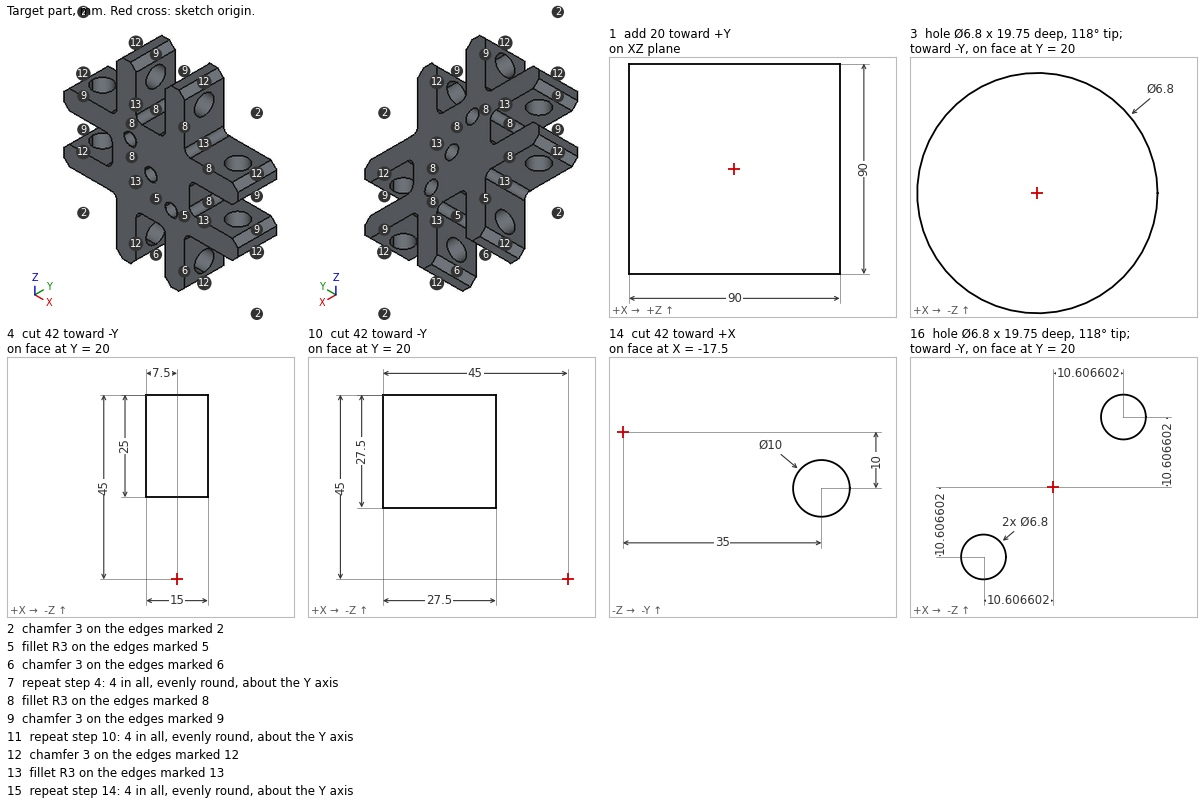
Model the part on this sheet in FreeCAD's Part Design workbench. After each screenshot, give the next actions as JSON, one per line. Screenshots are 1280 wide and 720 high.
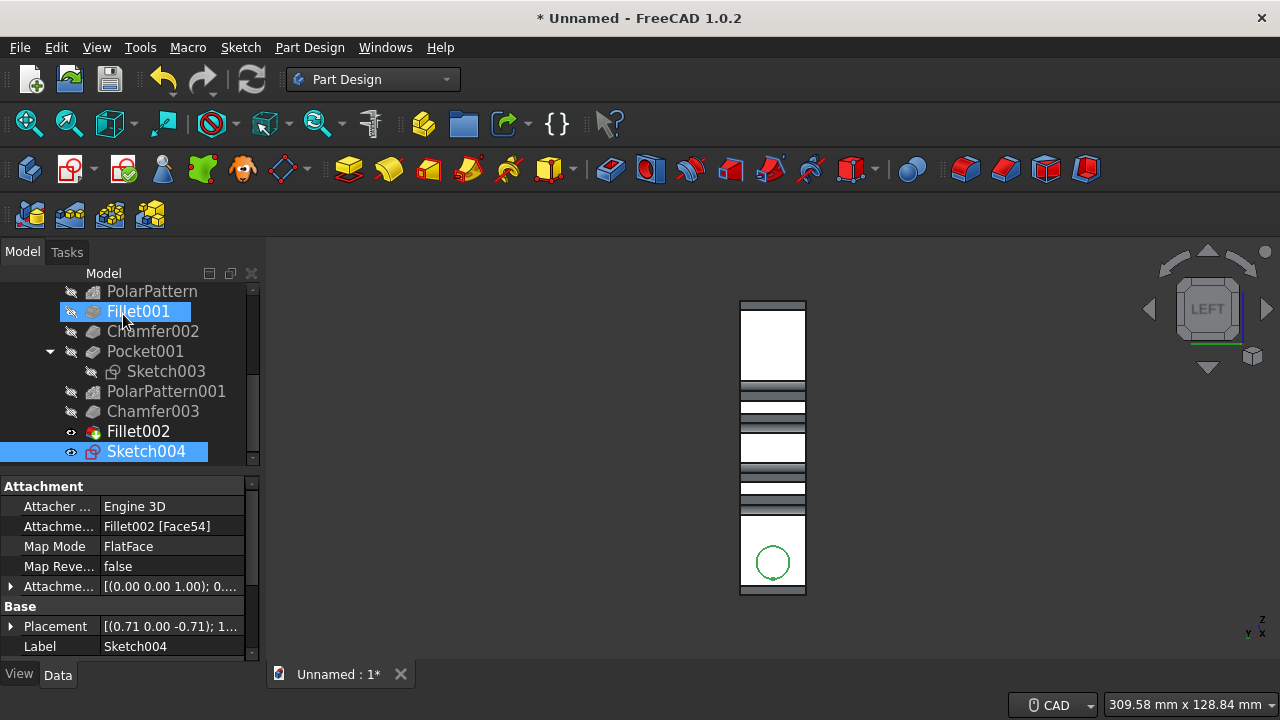
{"action": "left_click", "coordinate": [612, 170]}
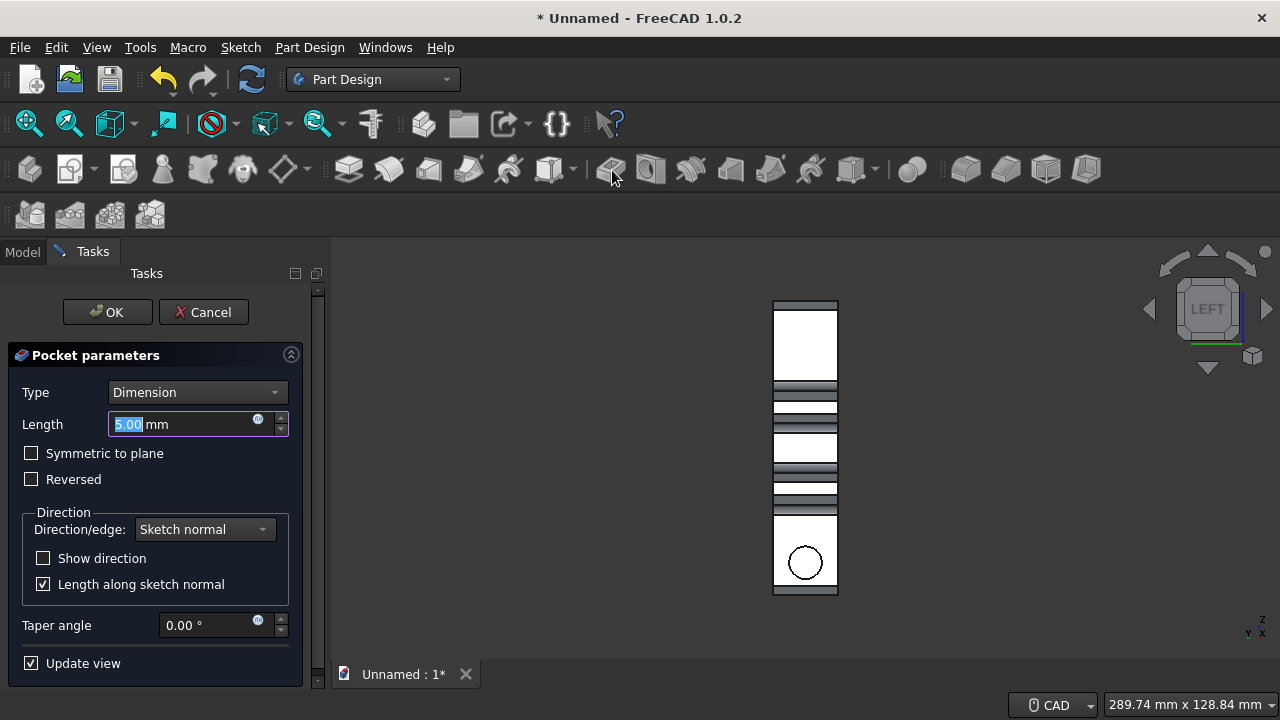
{"action": "type", "text": "42"}
{"action": "key", "text": "Tab"}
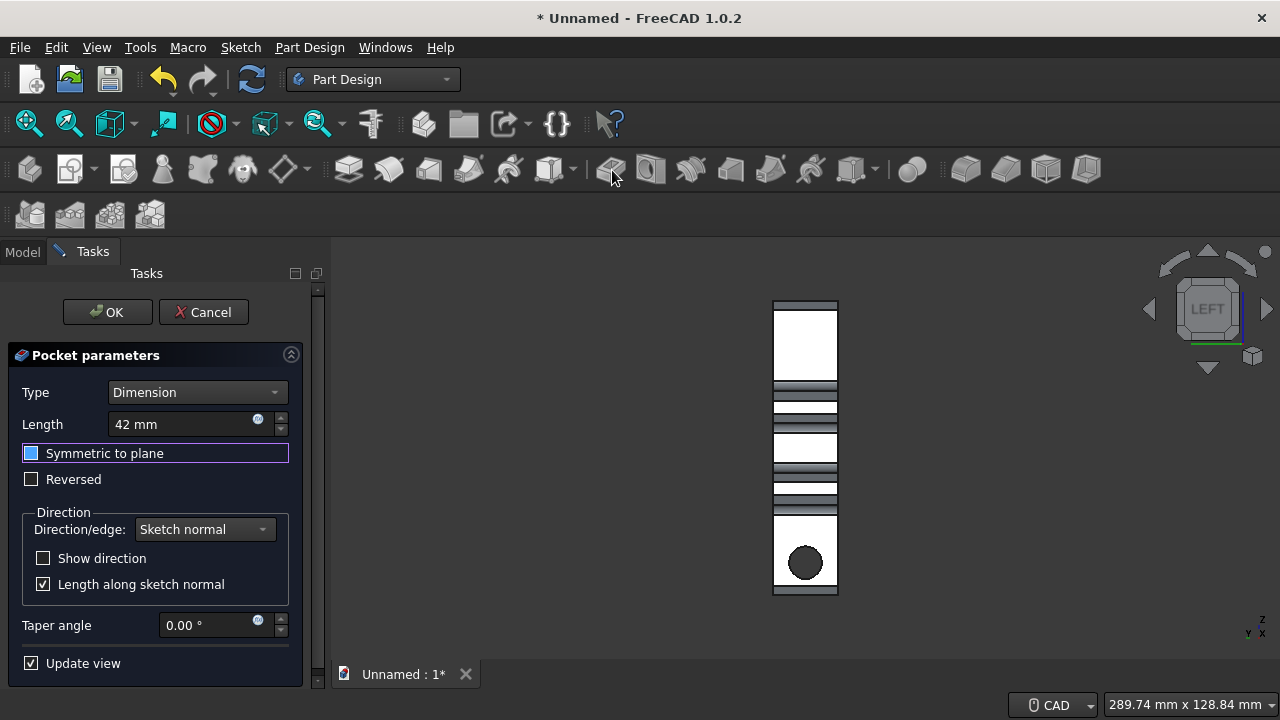
{"action": "left_click", "coordinate": [108, 312]}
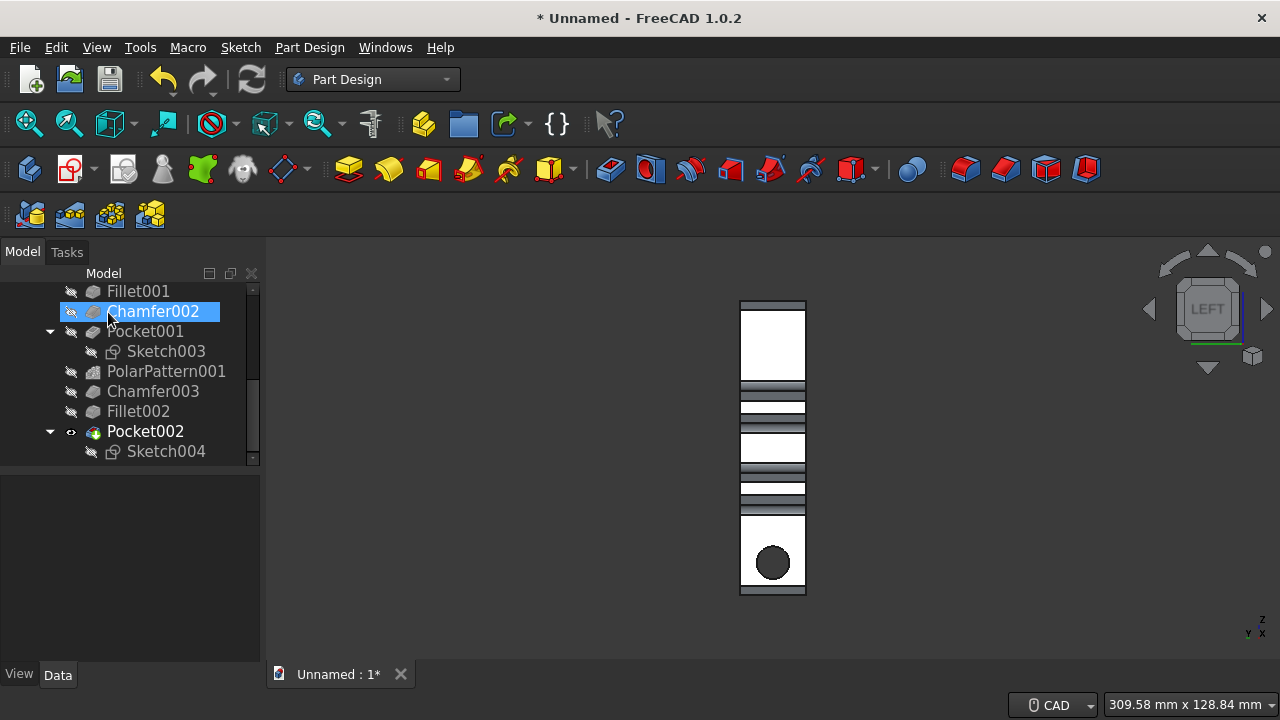
{"action": "left_click", "coordinate": [116, 432]}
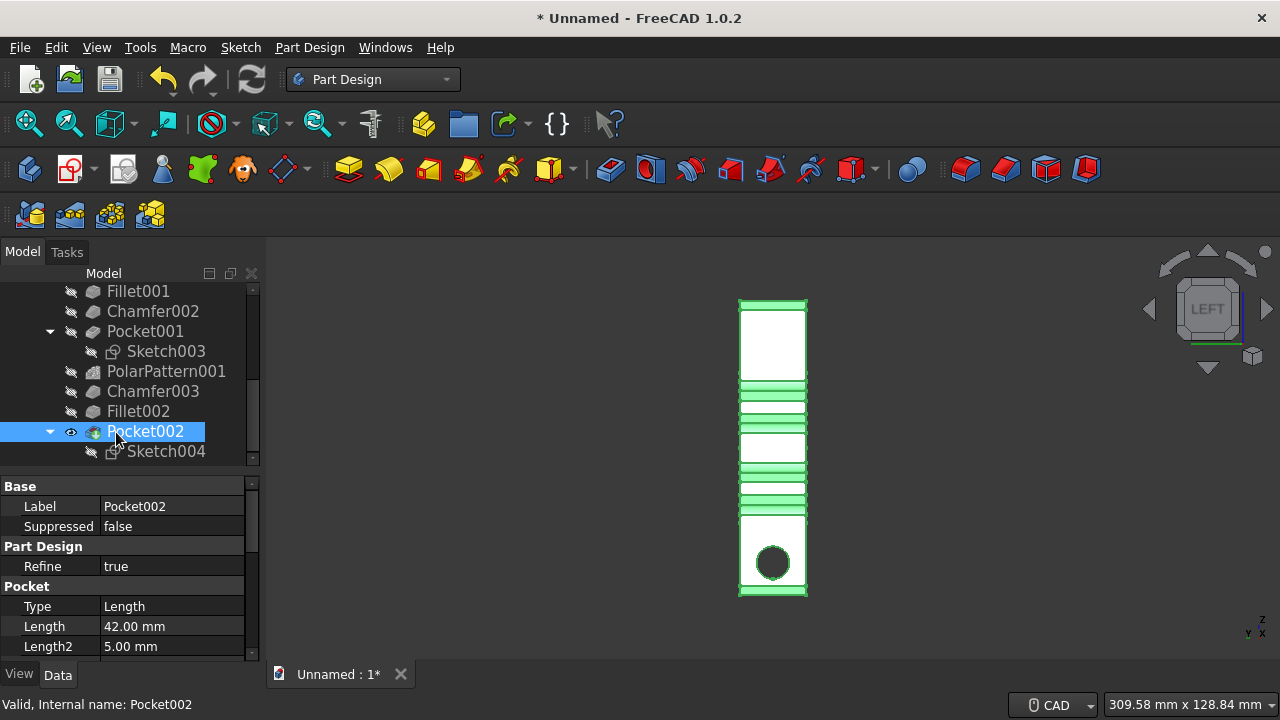
{"action": "left_click", "coordinate": [110, 214]}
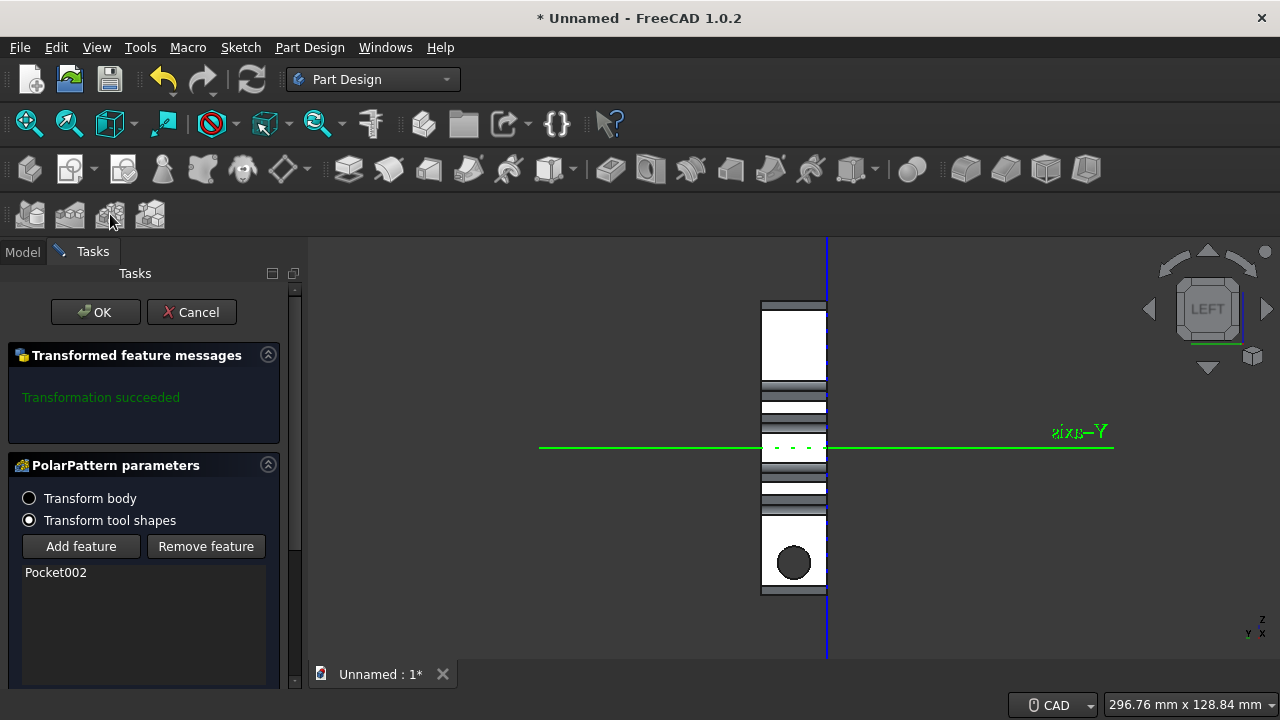
{"action": "scroll", "coordinate": [295, 486], "scroll_direction": "down", "scroll_amount": 2}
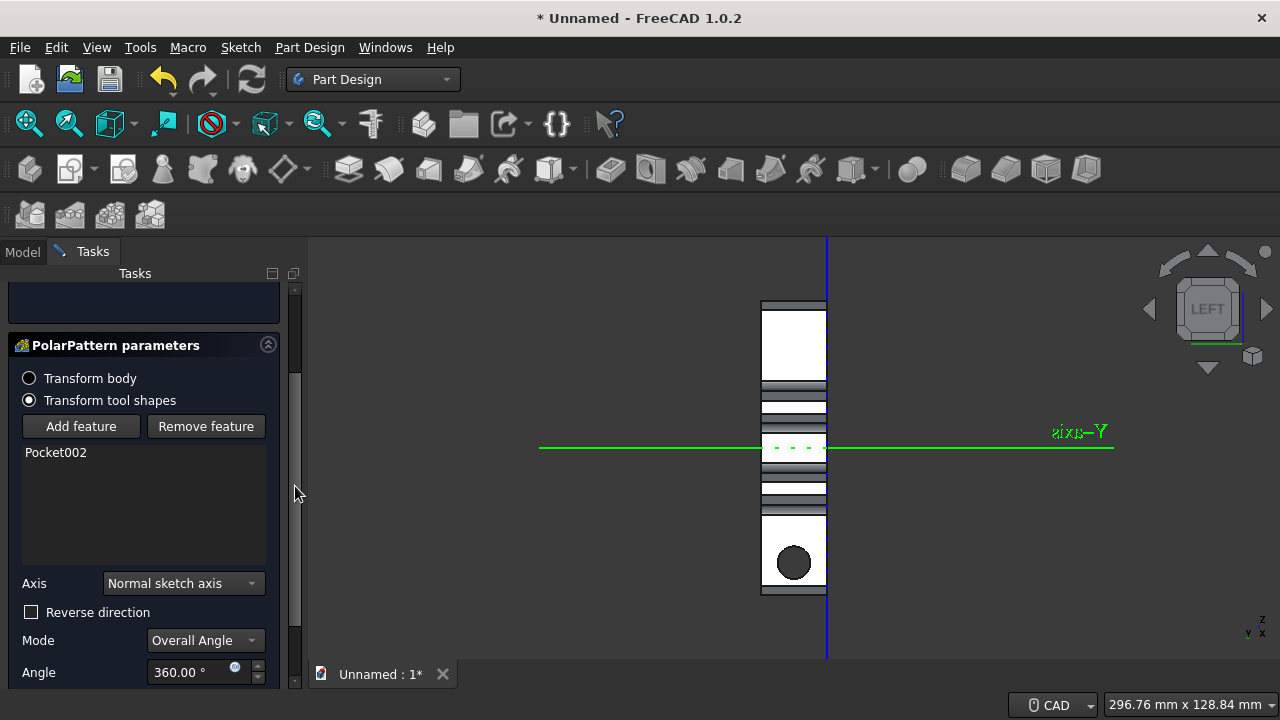
{"action": "left_click", "coordinate": [184, 584]}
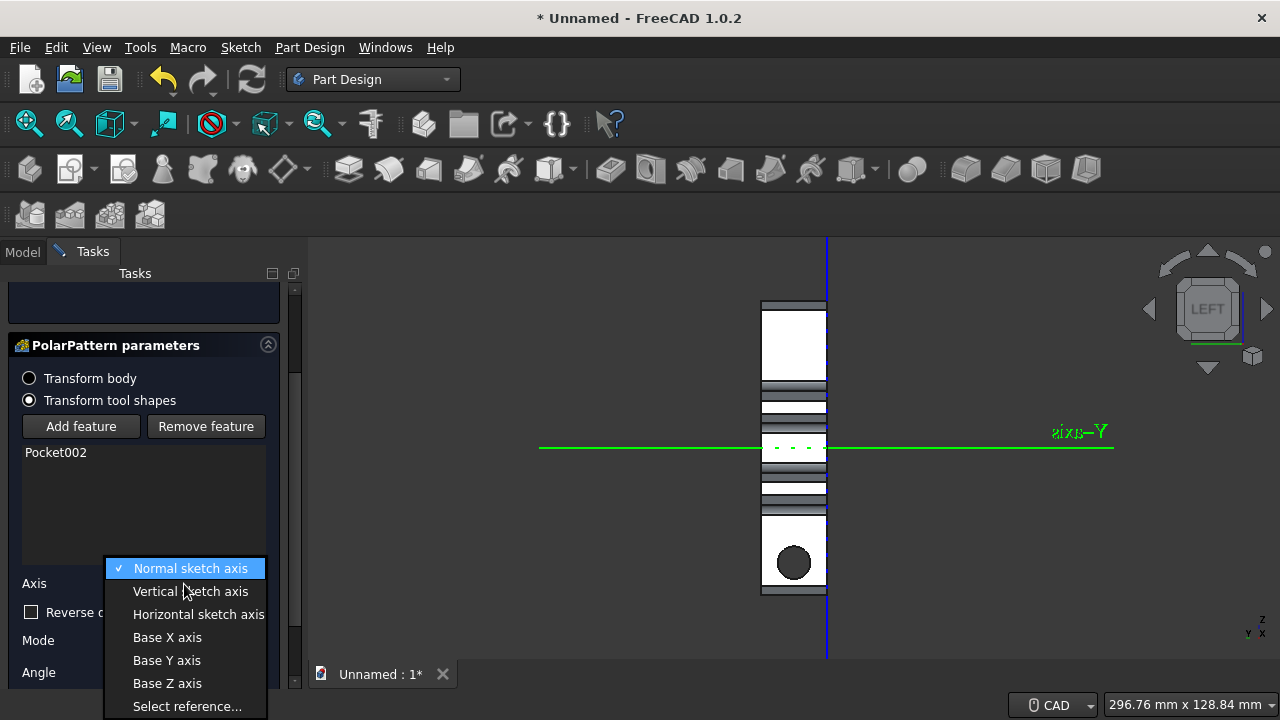
{"action": "left_click", "coordinate": [184, 660]}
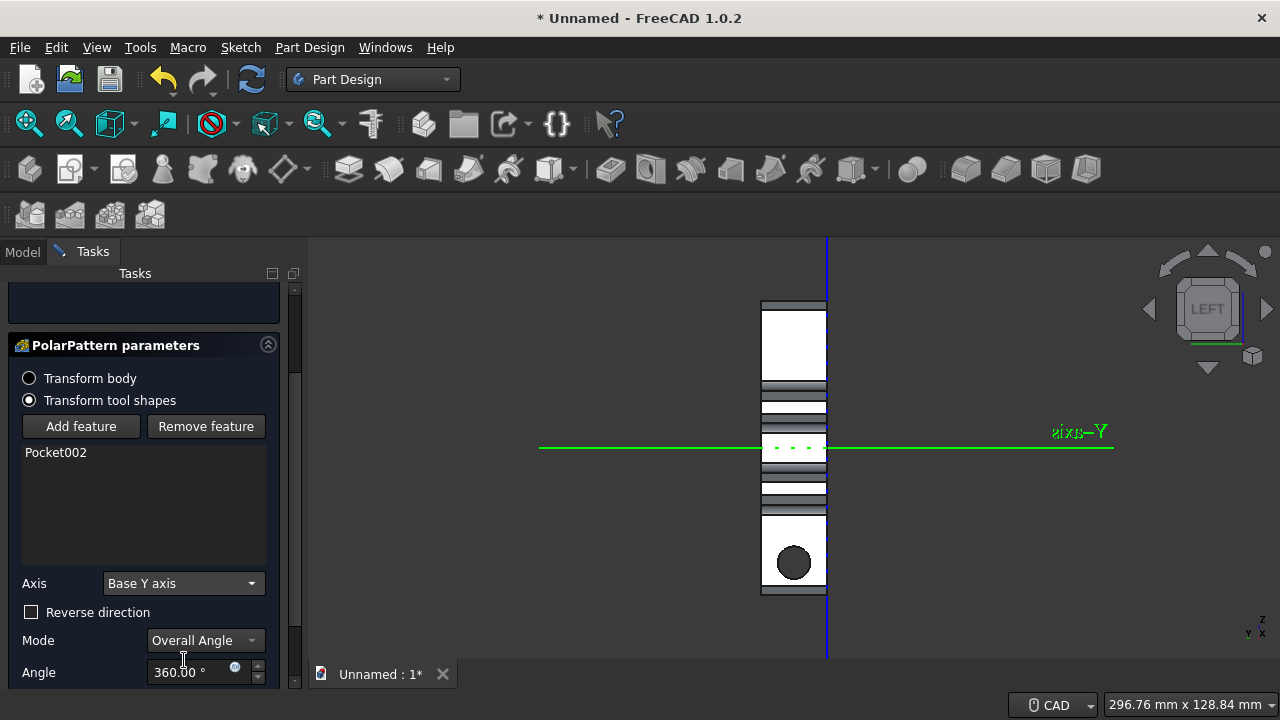
{"action": "scroll", "coordinate": [295, 486], "scroll_direction": "down", "scroll_amount": 2}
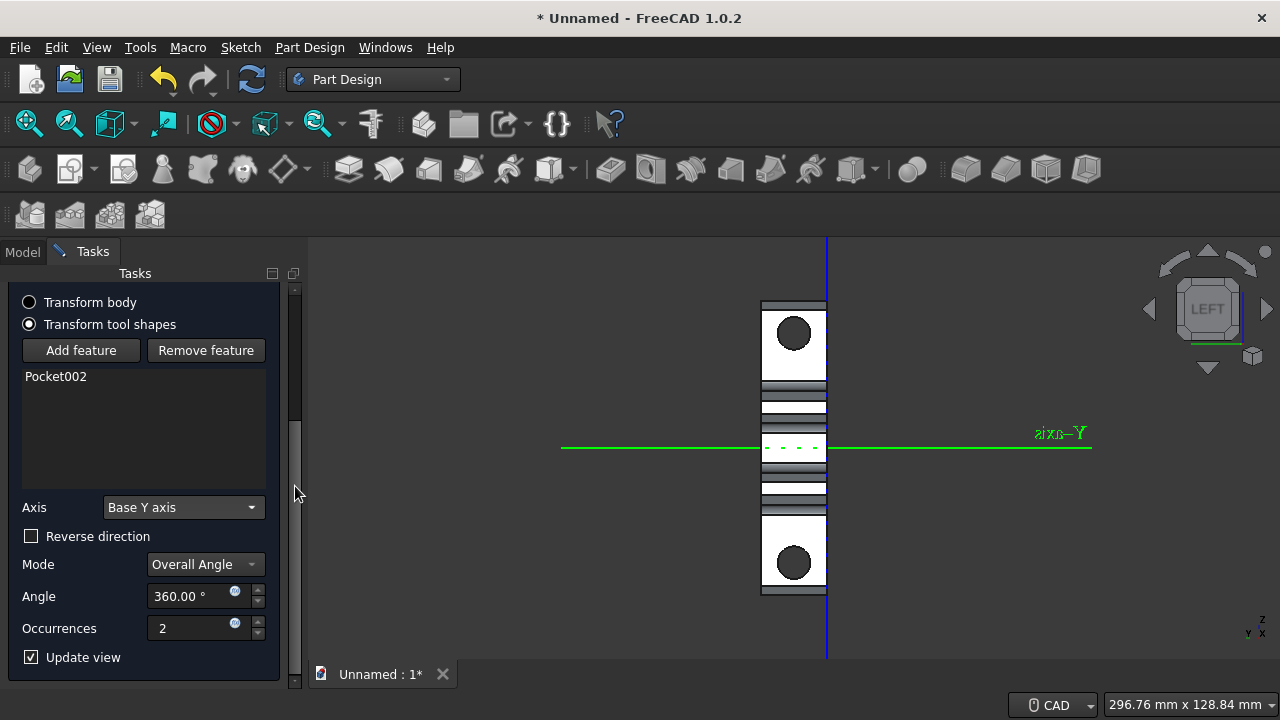
{"action": "triple_click", "coordinate": [198, 628]}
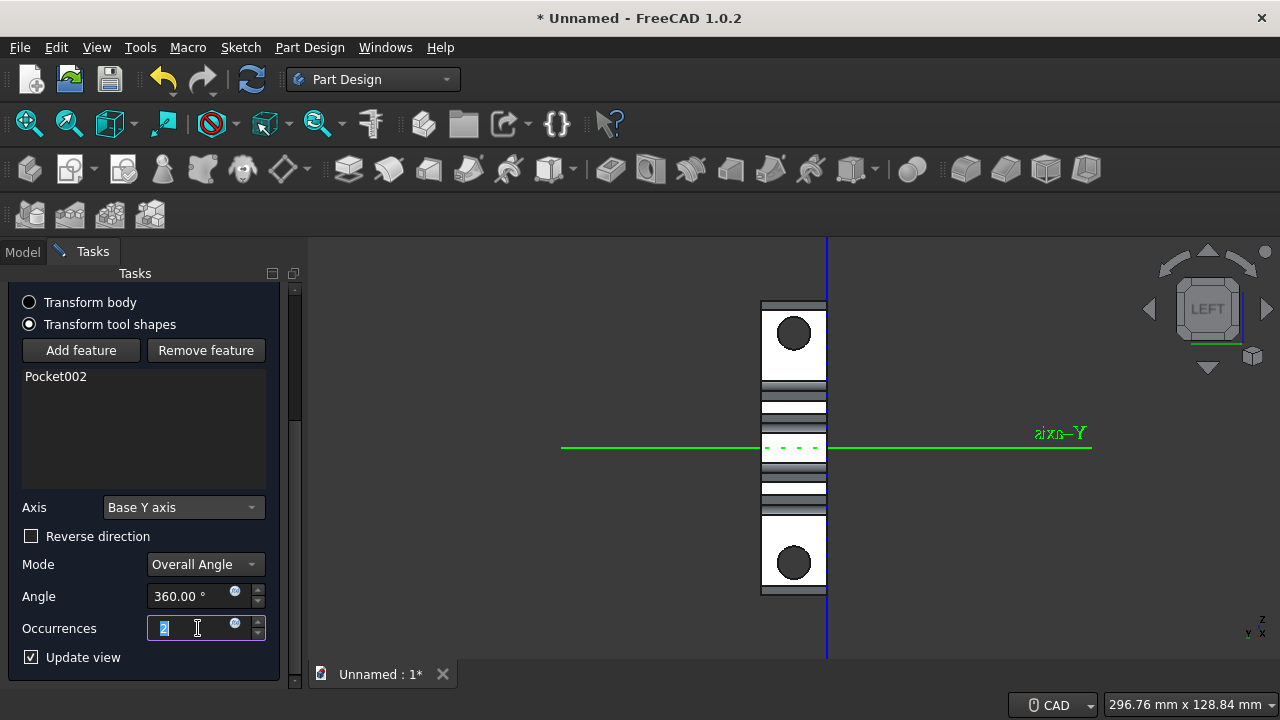
{"action": "type", "text": "4"}
{"action": "key", "text": "Tab"}